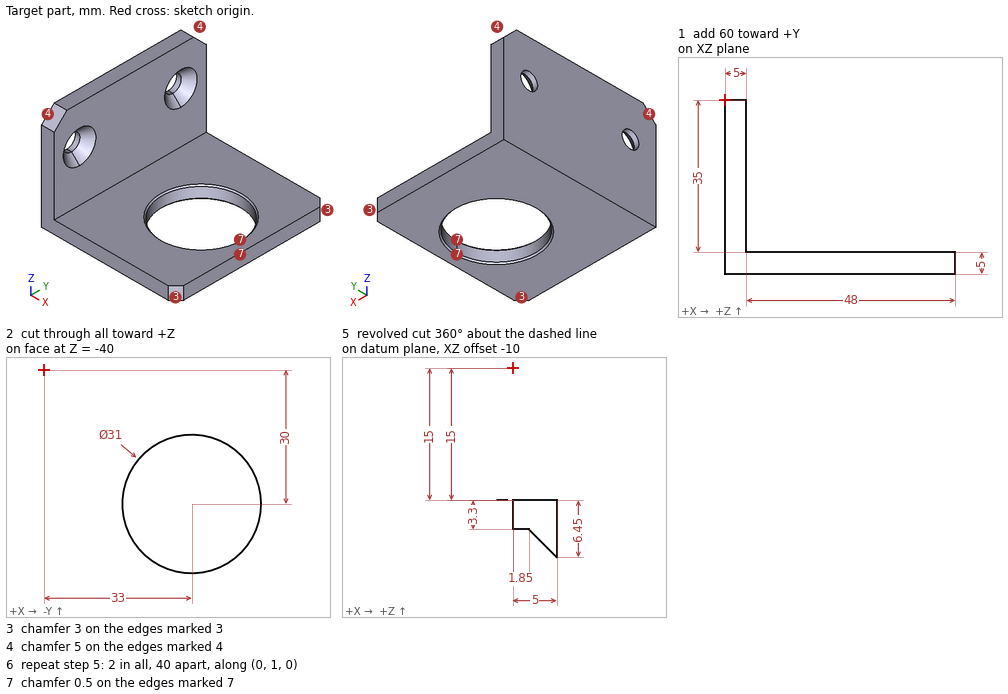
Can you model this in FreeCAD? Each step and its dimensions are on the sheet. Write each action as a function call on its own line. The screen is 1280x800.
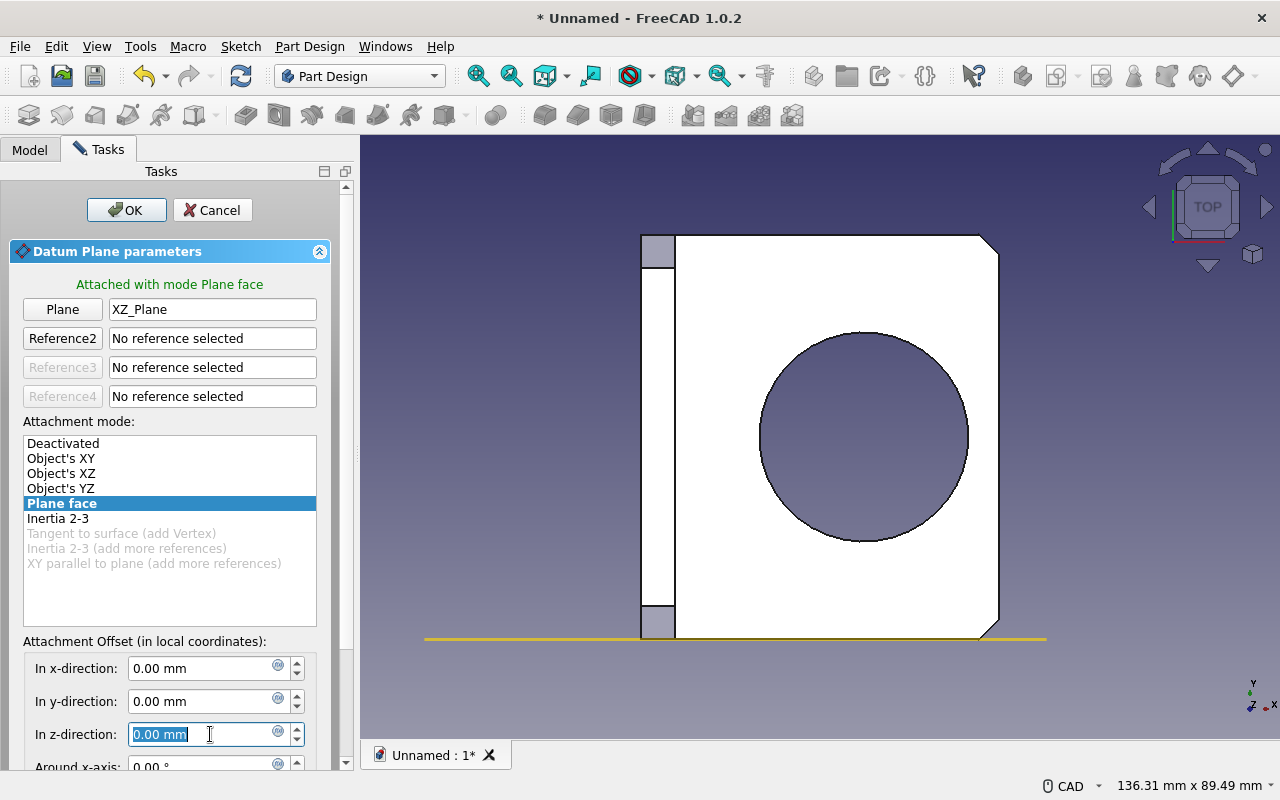
text(-10)
key(Tab)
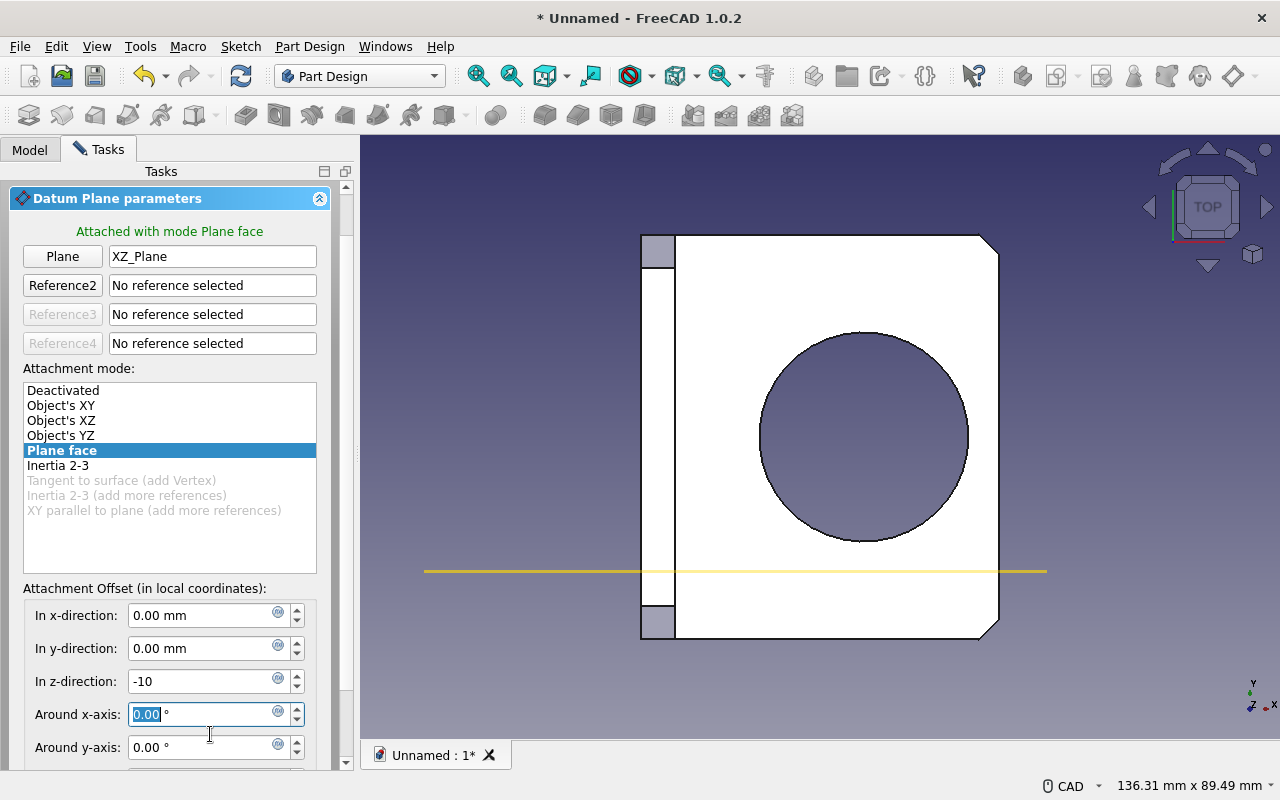
scroll(346, 476, up, 2)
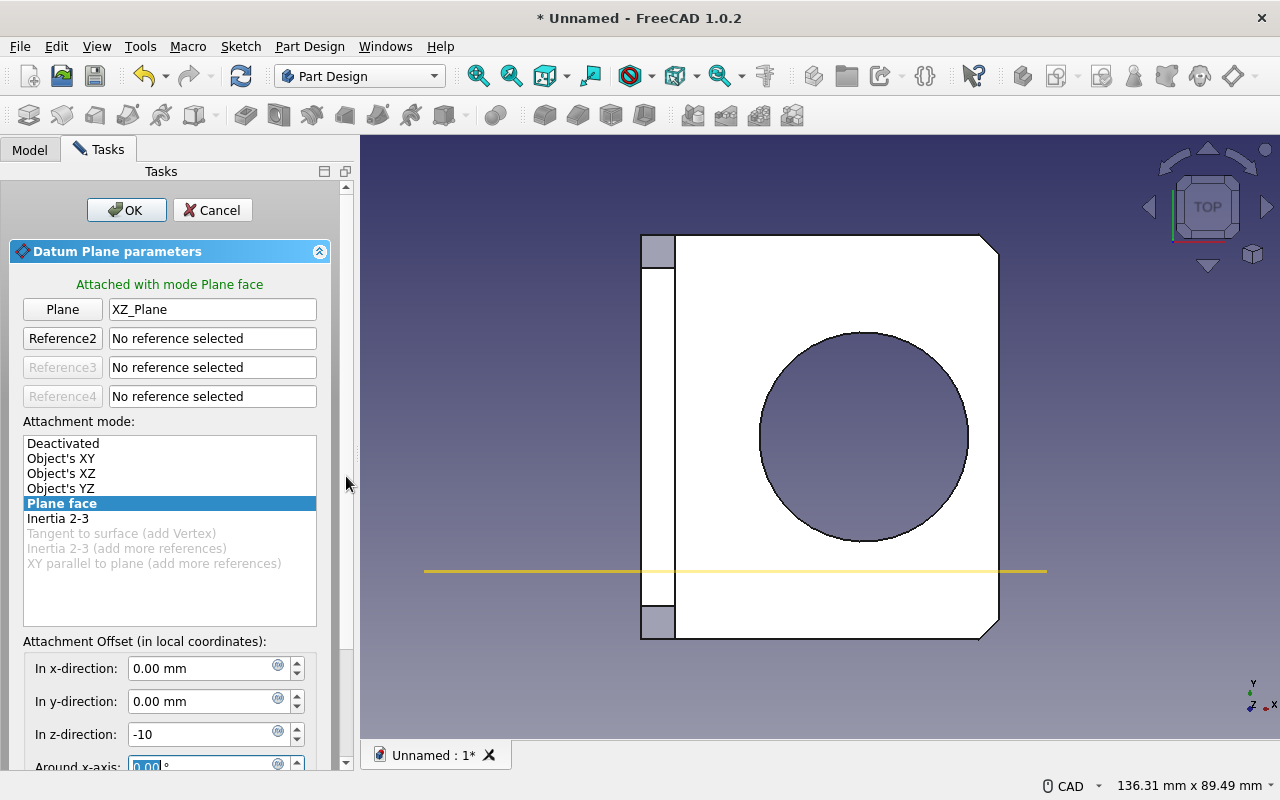
click(127, 210)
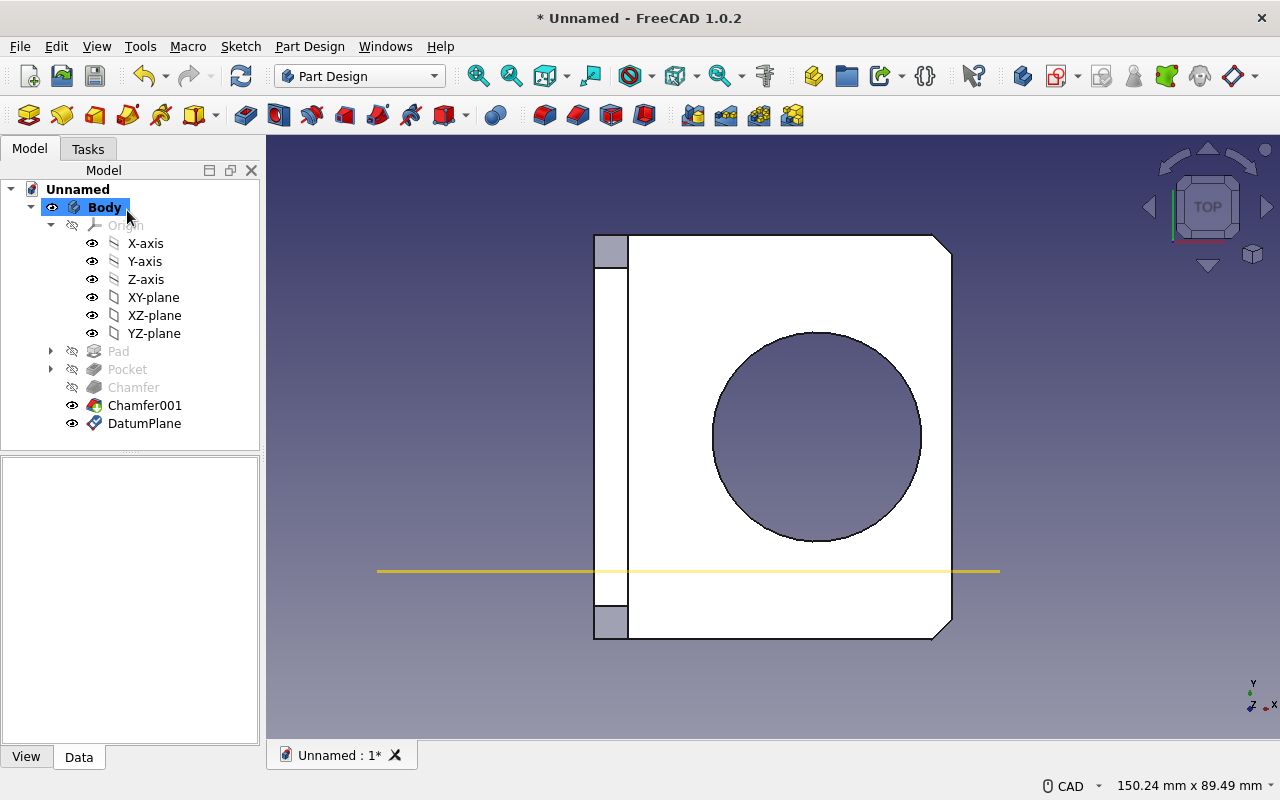
click(117, 423)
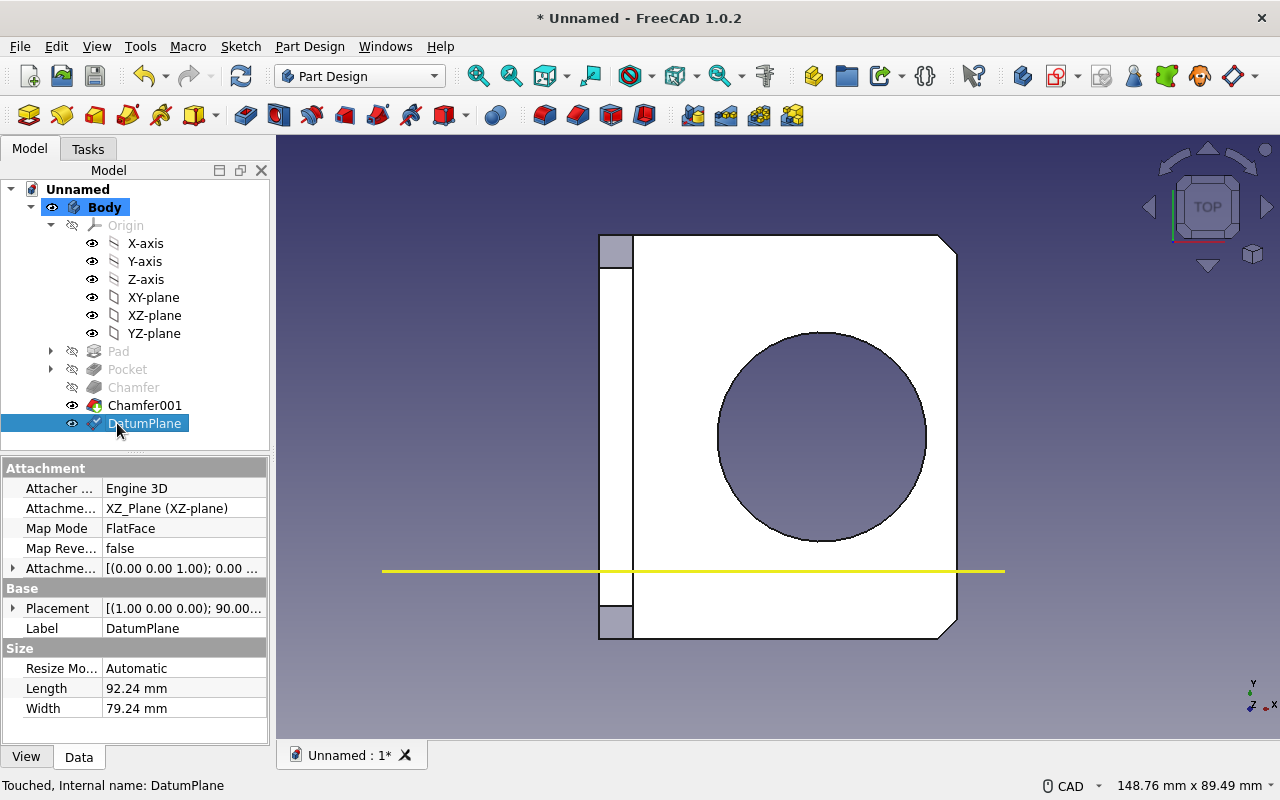
click(1056, 76)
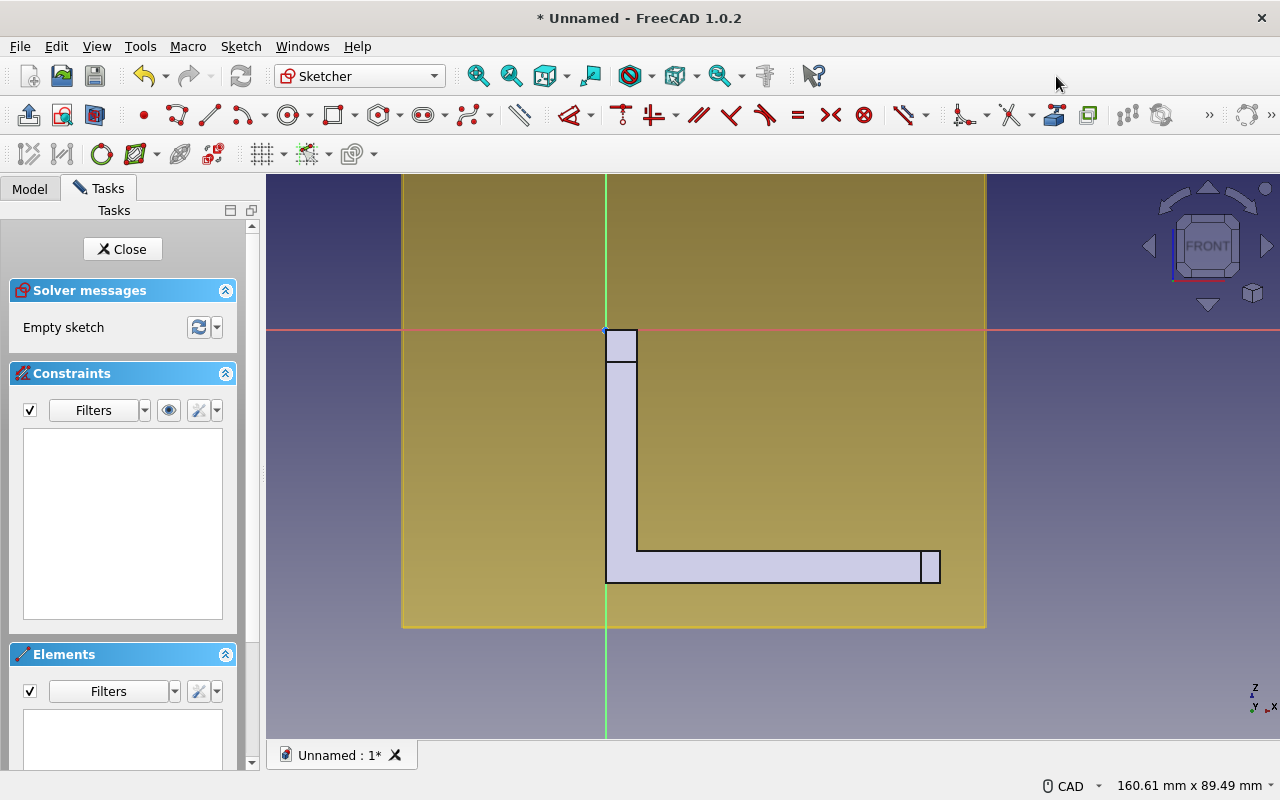
click(95, 116)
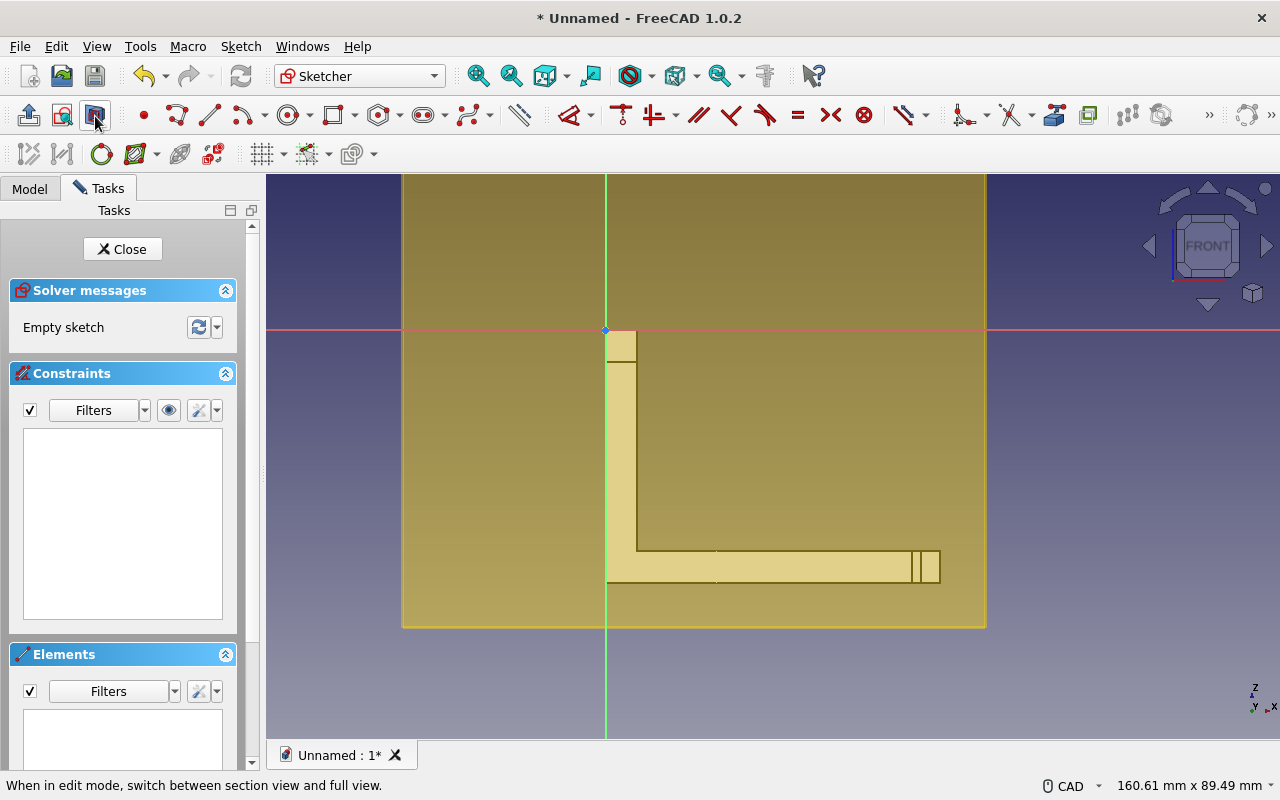
scroll(604, 444, up, 11)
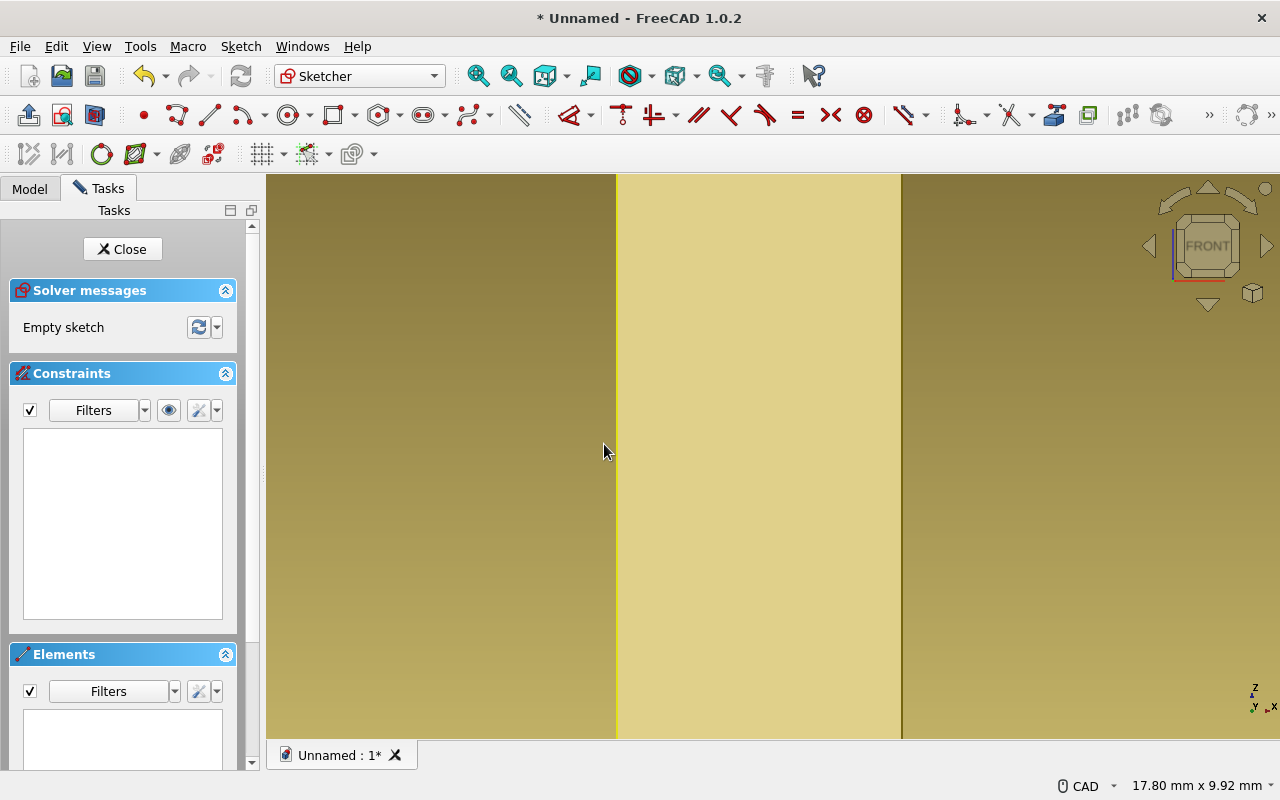
click(177, 116)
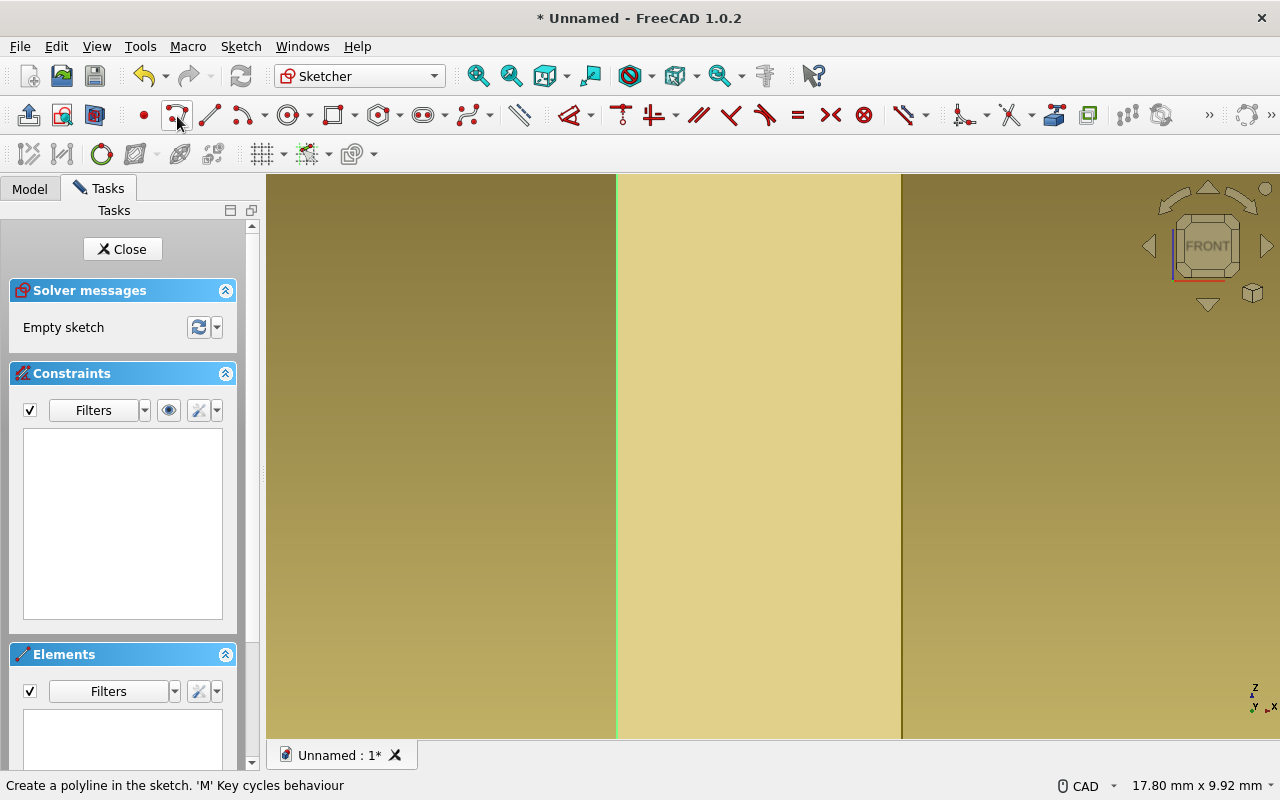
click(617, 268)
click(902, 268)
click(902, 636)
click(722, 456)
click(626, 456)
click(617, 269)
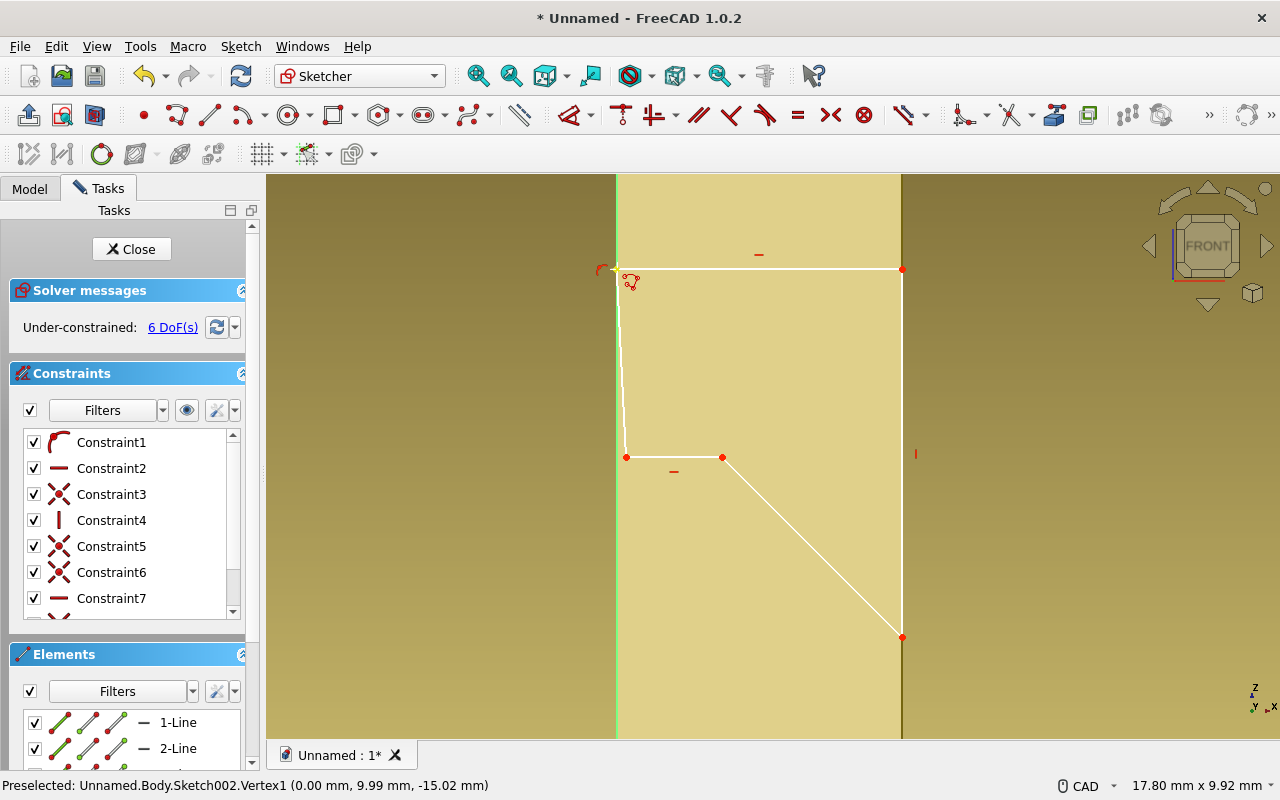
key(g)
key(l)